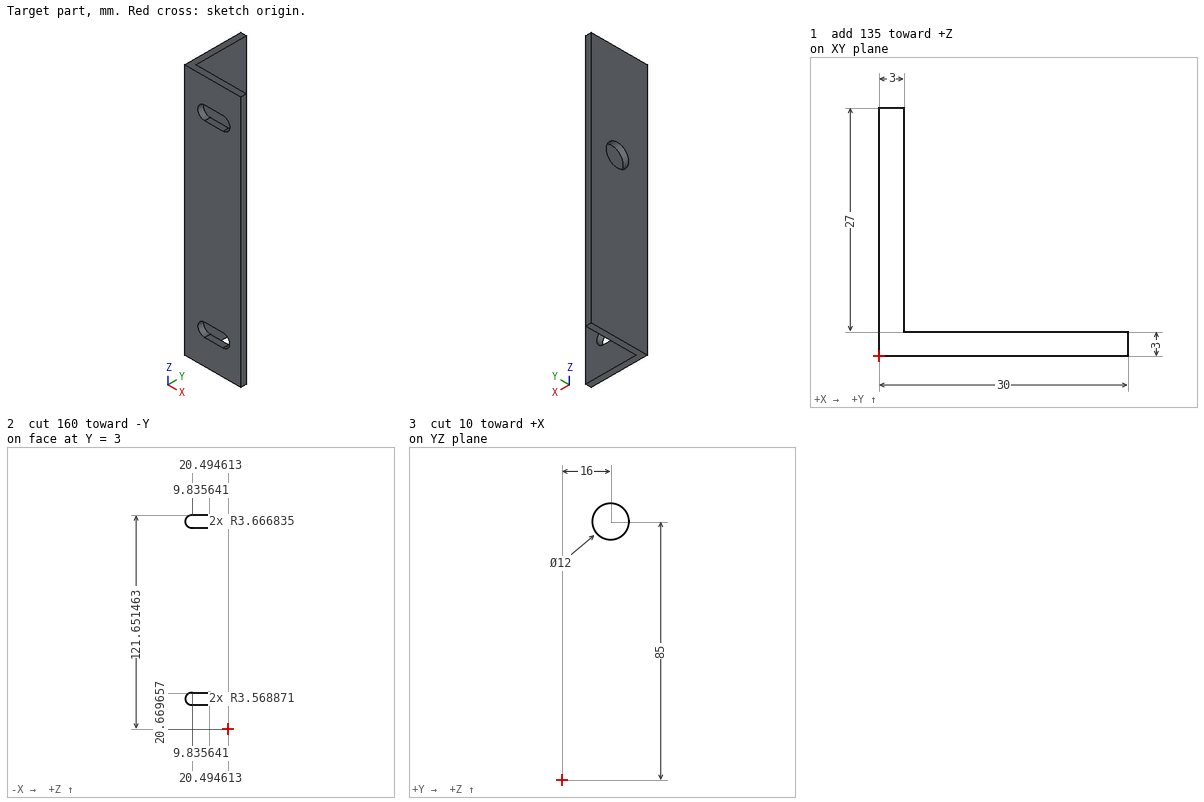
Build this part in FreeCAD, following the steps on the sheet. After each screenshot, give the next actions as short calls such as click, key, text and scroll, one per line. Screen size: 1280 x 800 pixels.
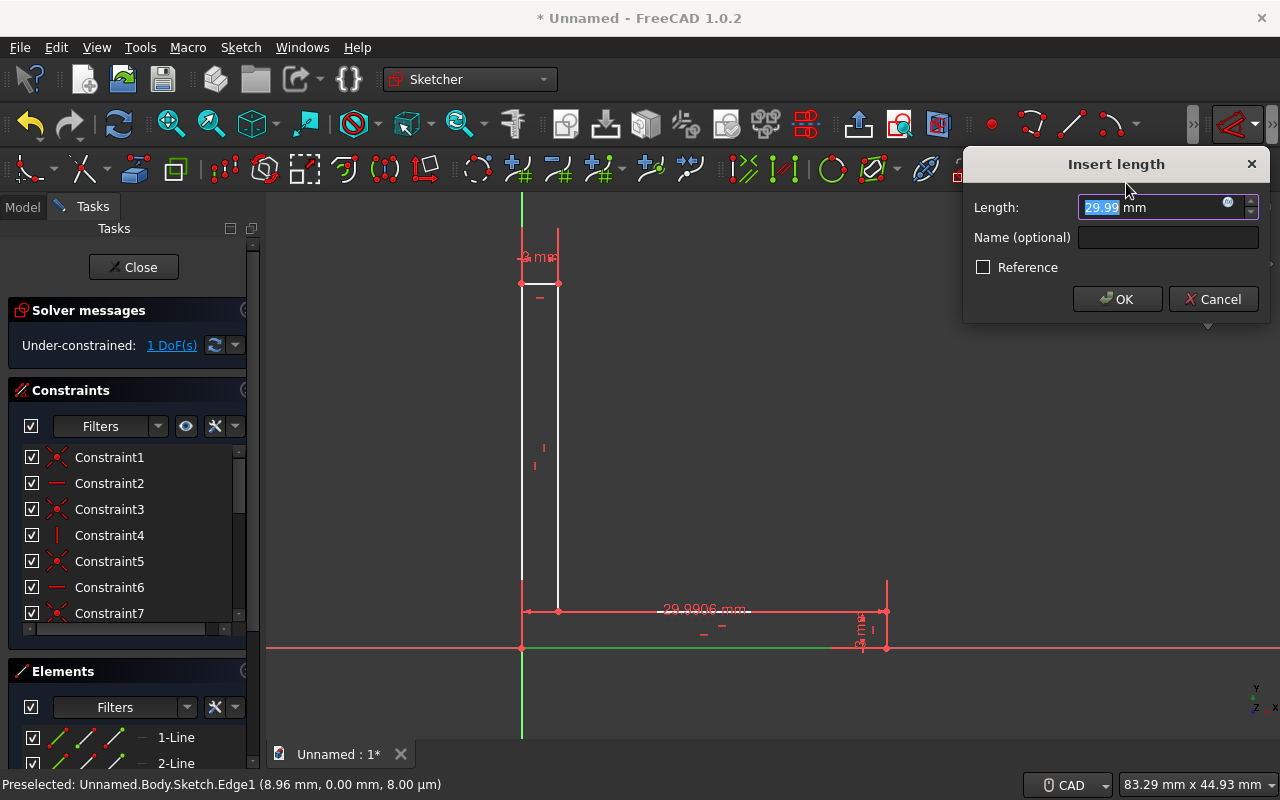
text(30)
key(Return)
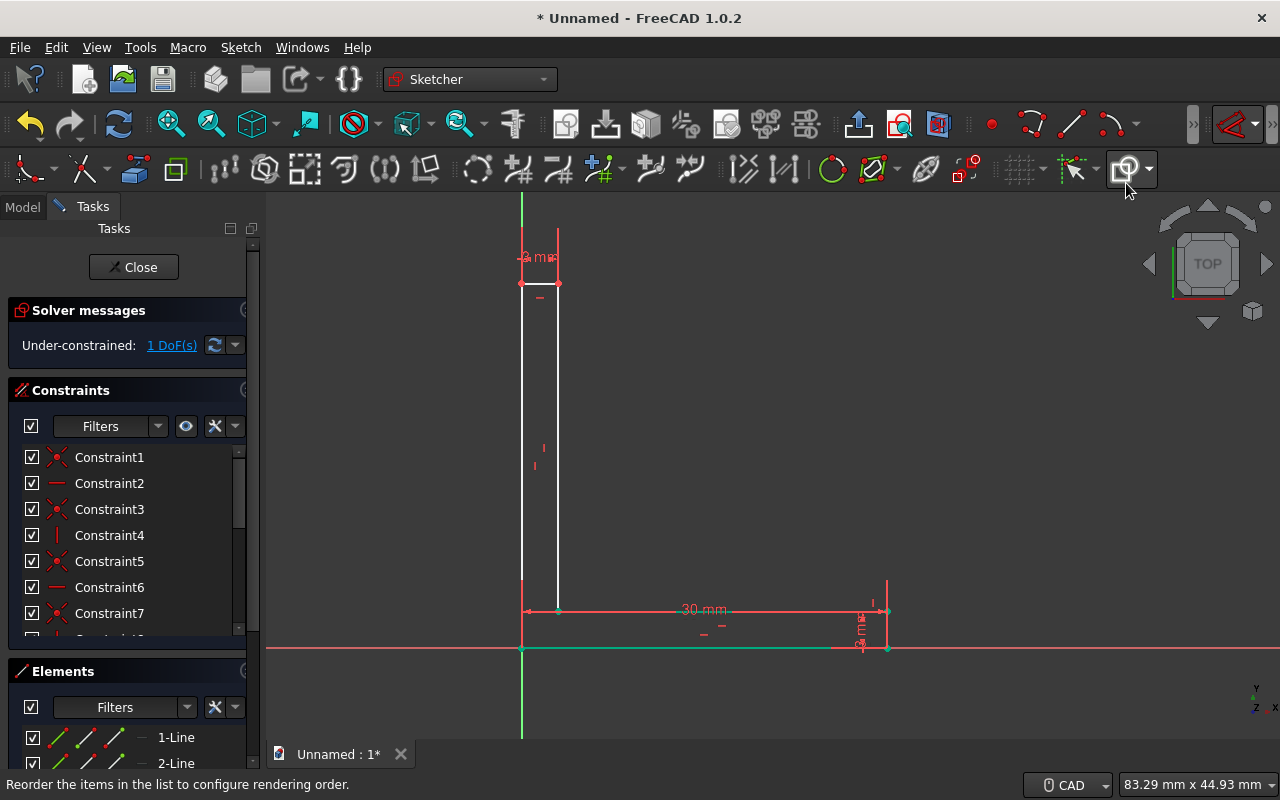
click(558, 513)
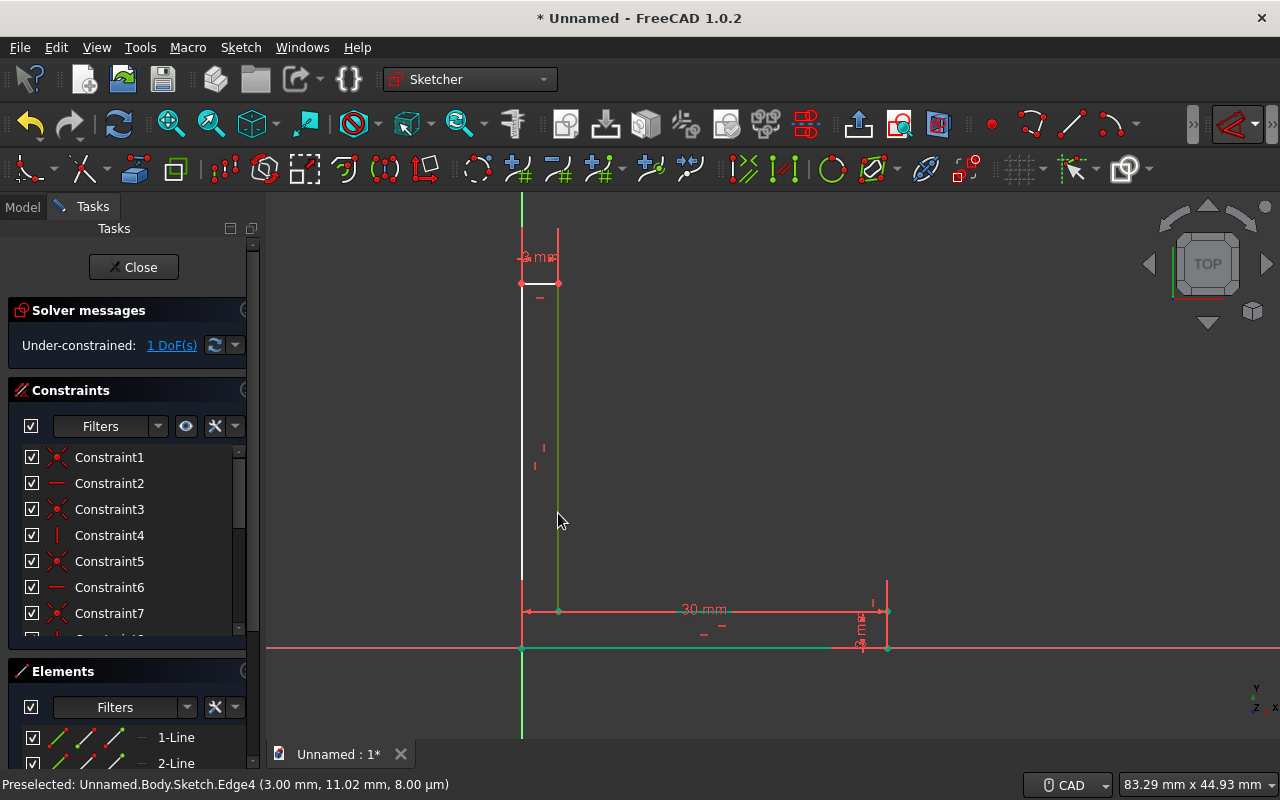
key(i)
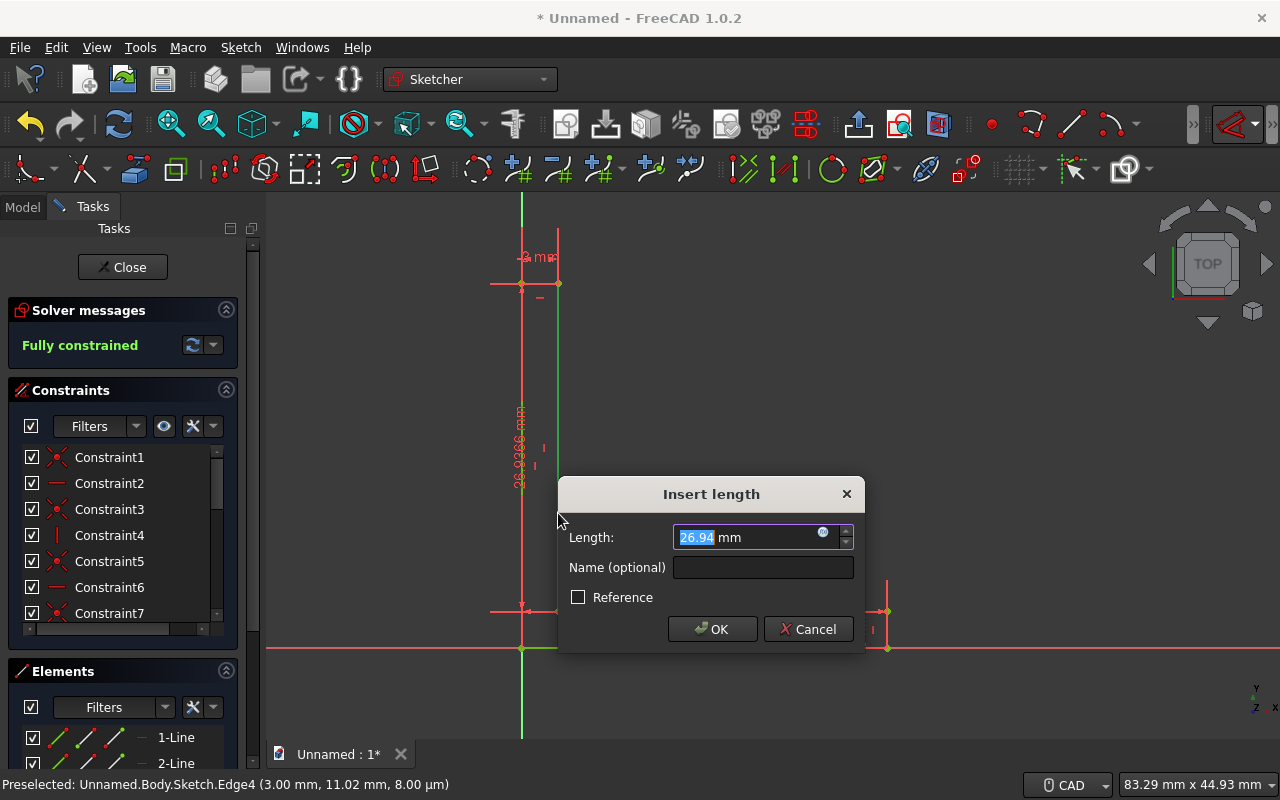
text(27)
key(Return)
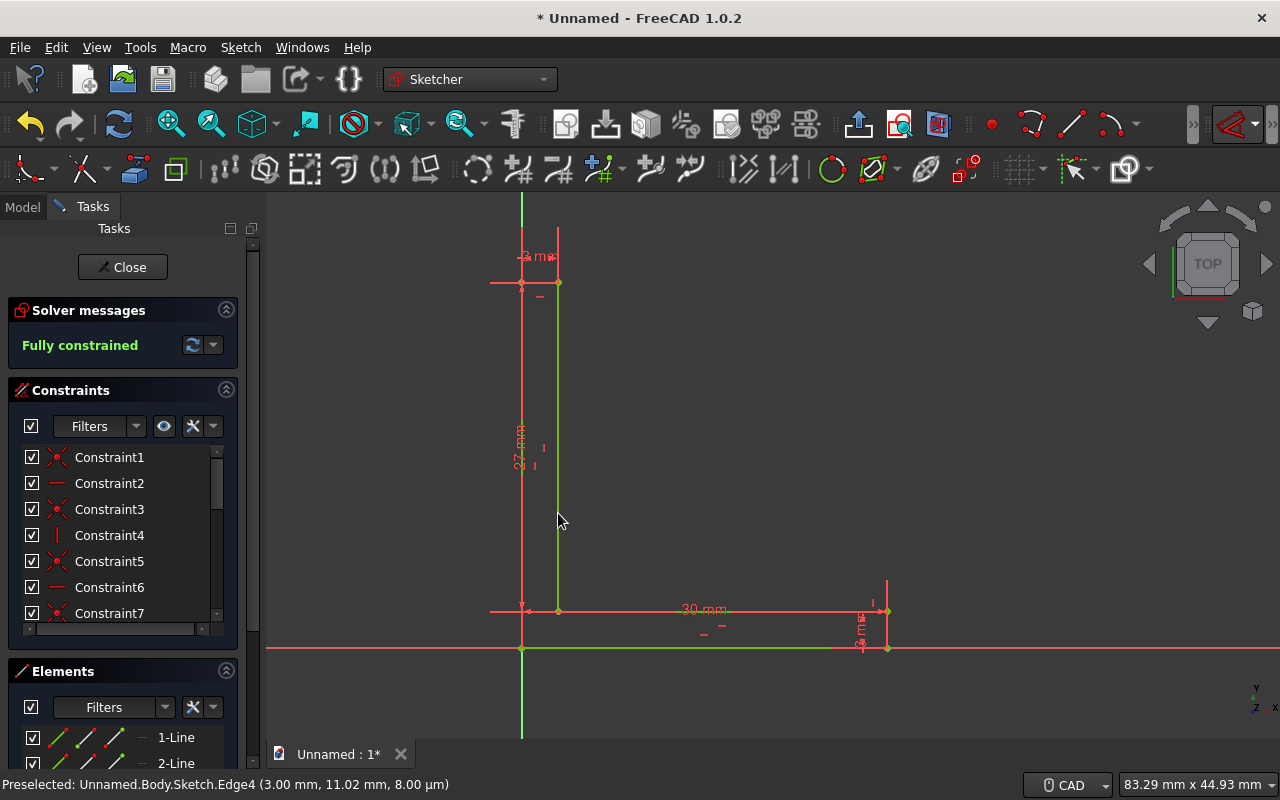
click(123, 267)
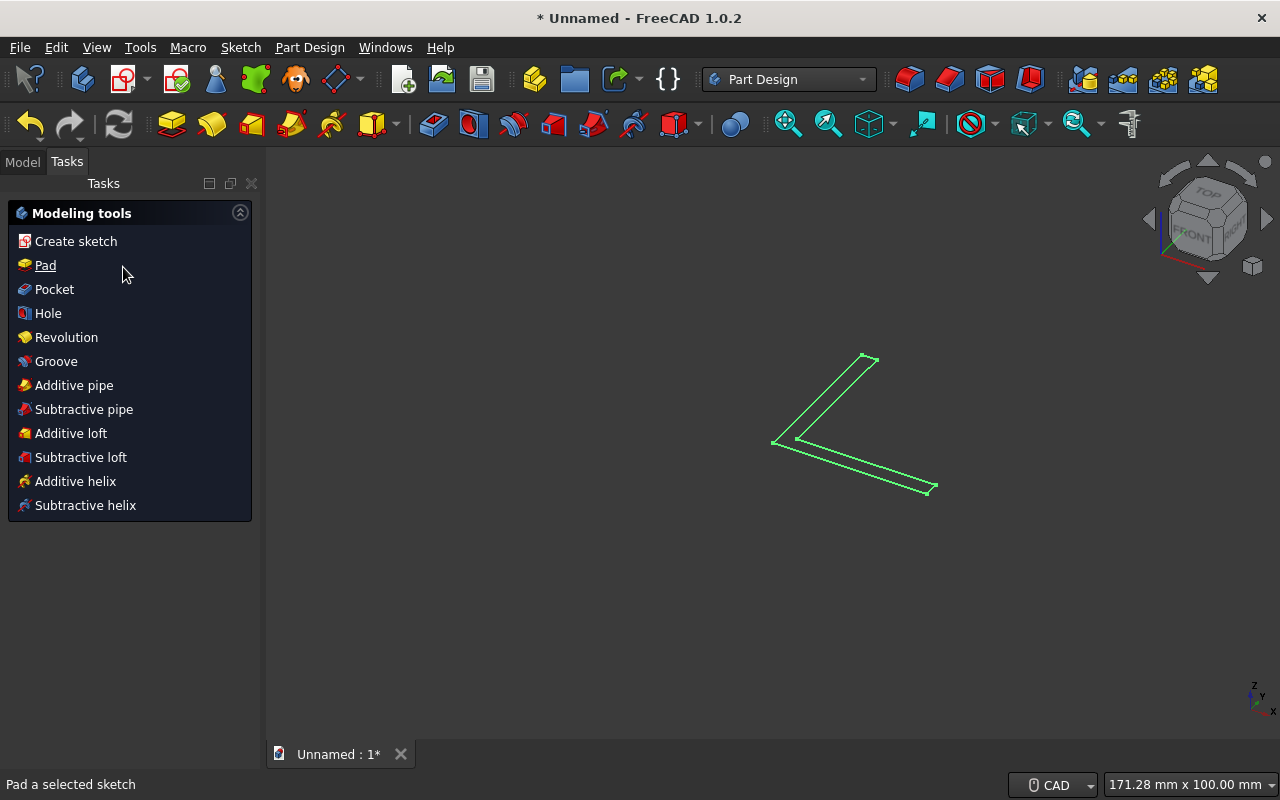
click(172, 124)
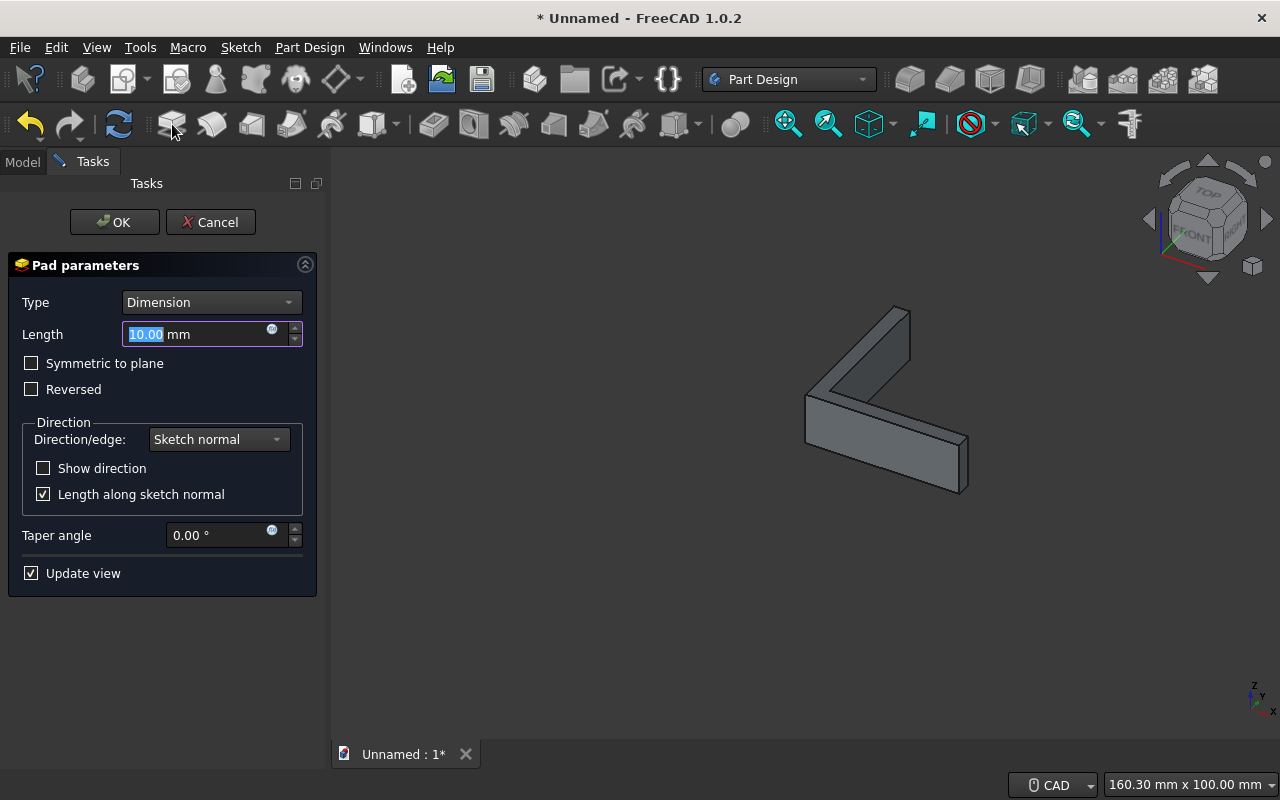
text(135)
key(Tab)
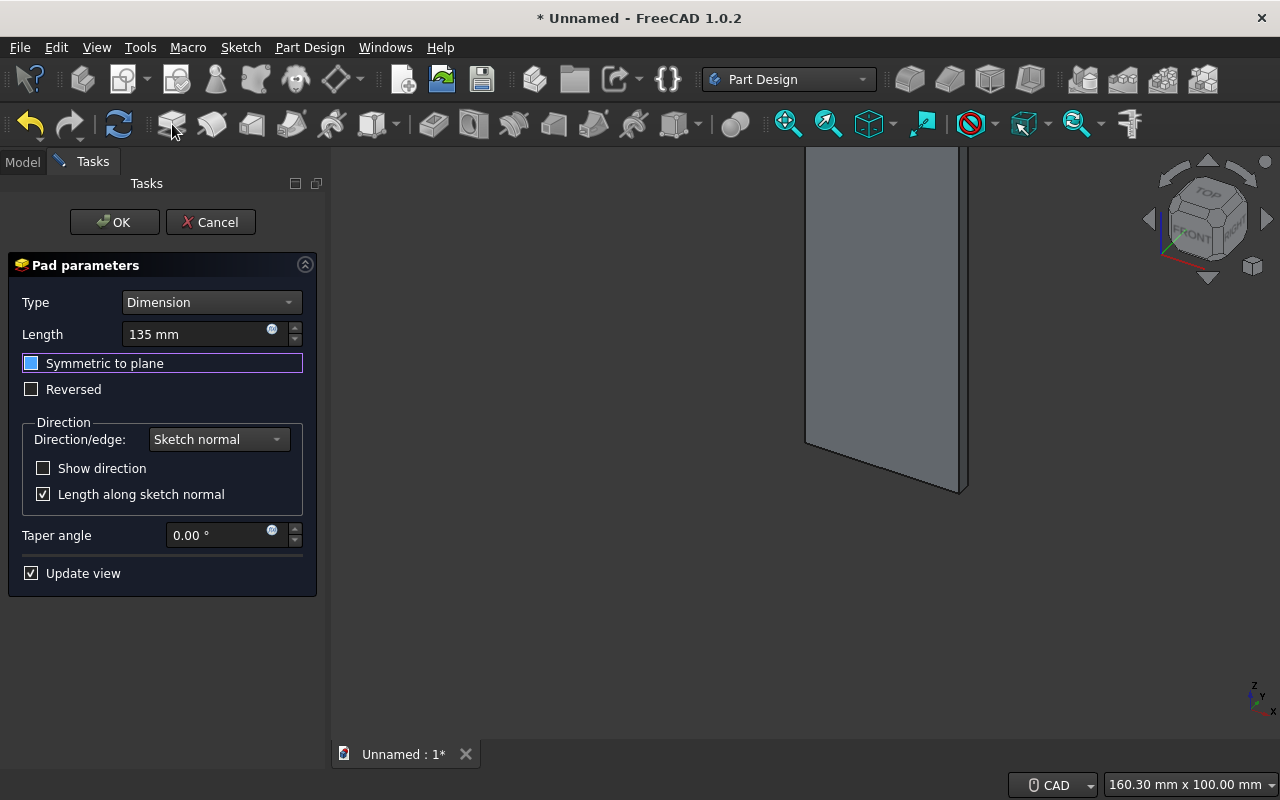
click(115, 222)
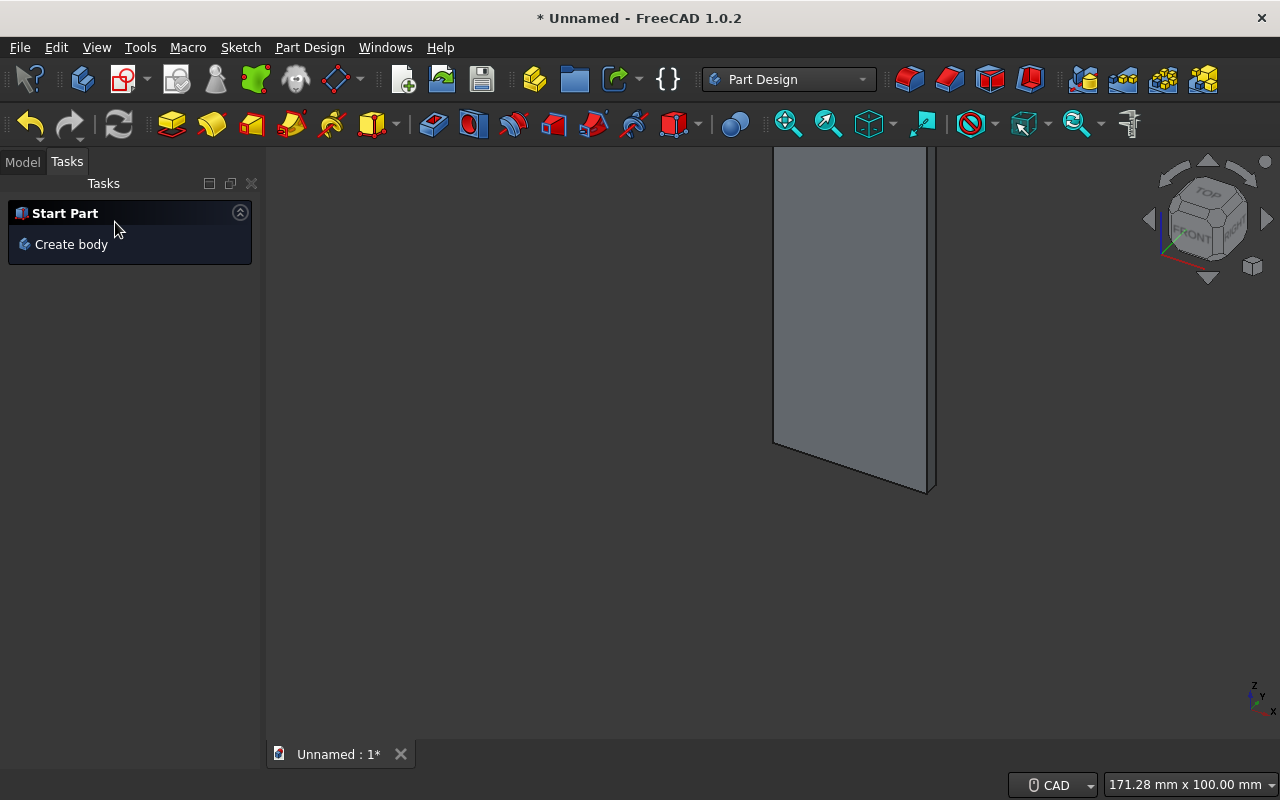
key(v)
key(f)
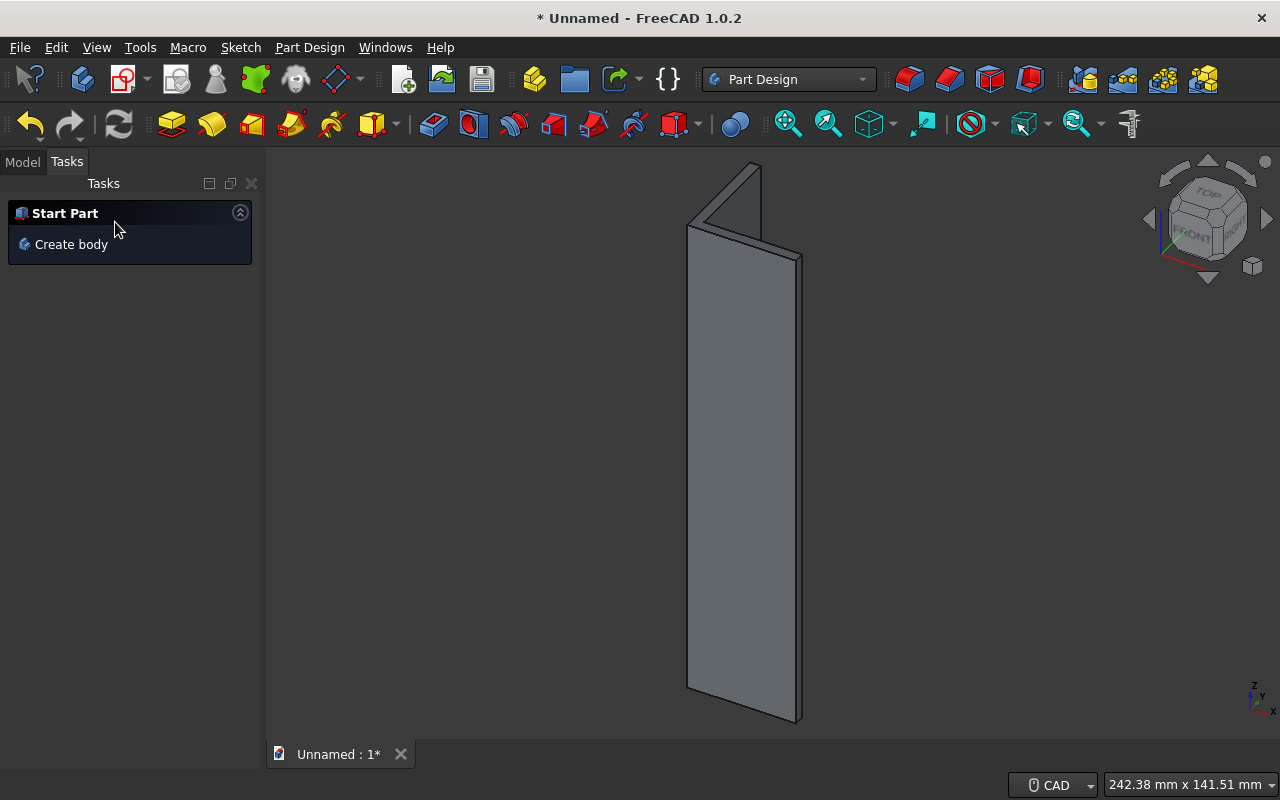
key(4)